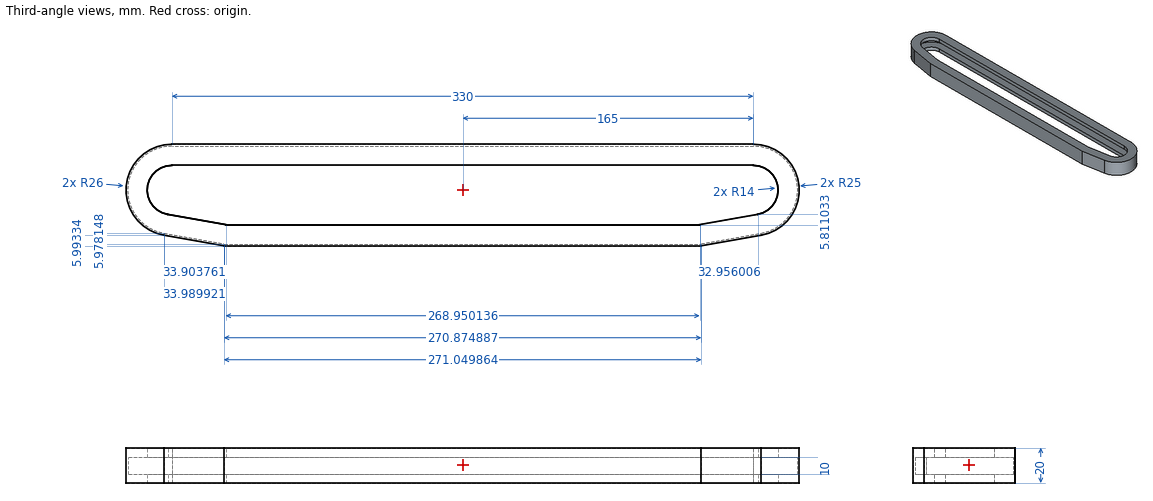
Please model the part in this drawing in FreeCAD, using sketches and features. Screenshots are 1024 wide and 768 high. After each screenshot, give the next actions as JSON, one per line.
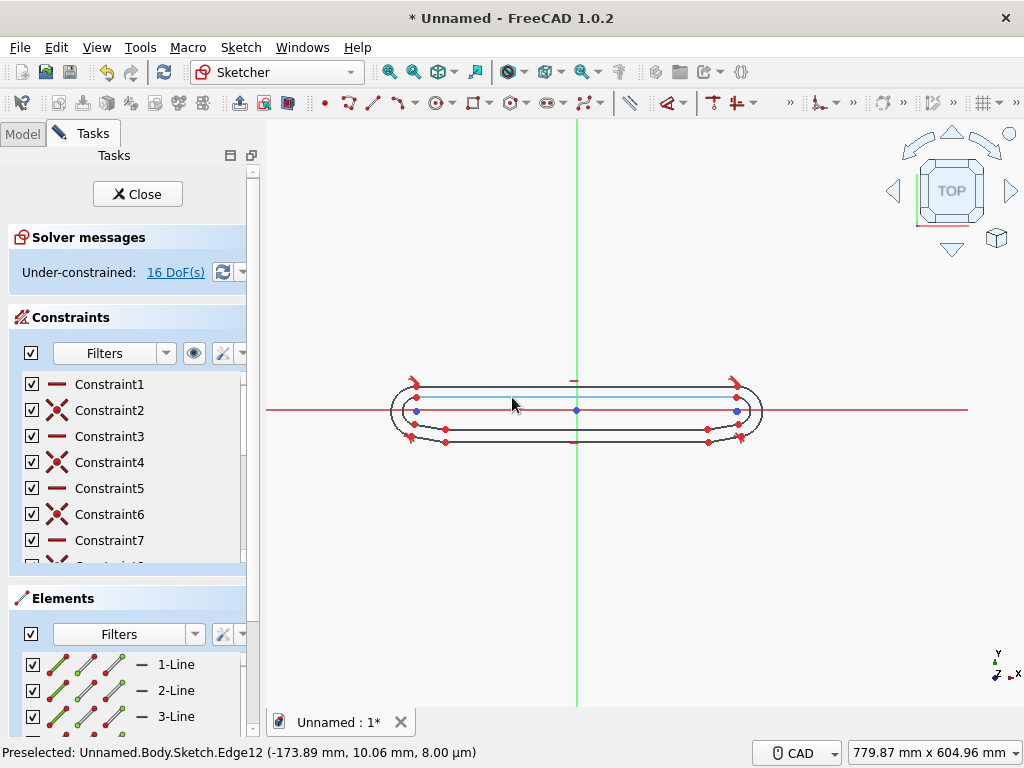
{"action": "left_click", "coordinate": [759, 424]}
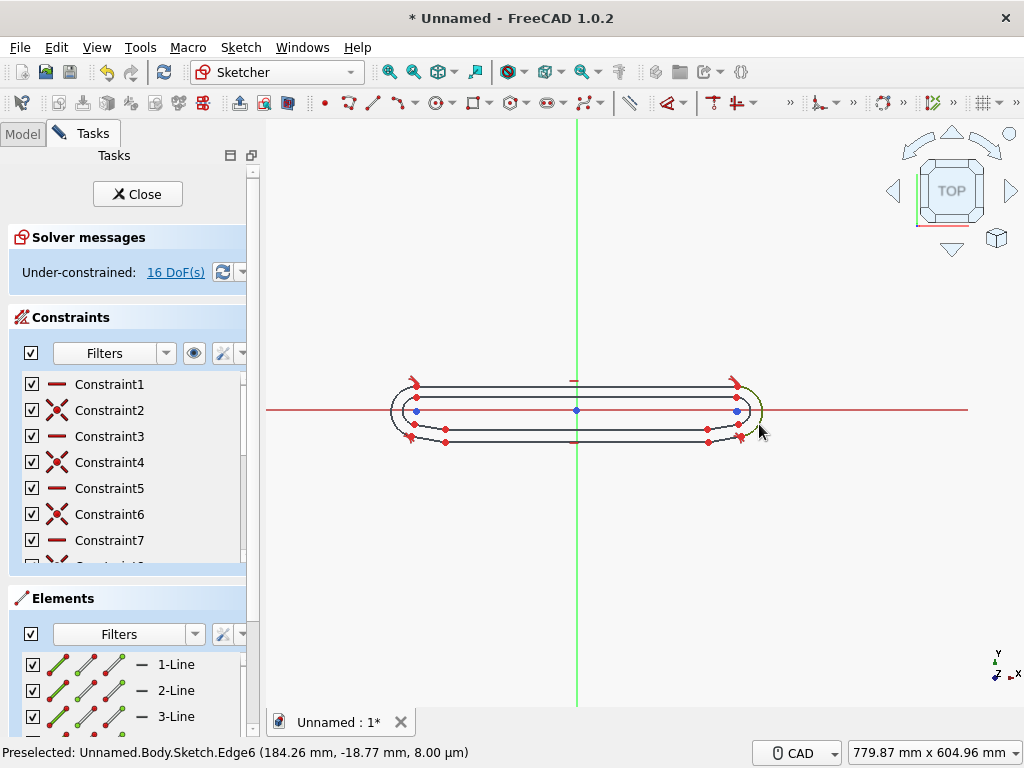
{"action": "left_click", "coordinate": [750, 410]}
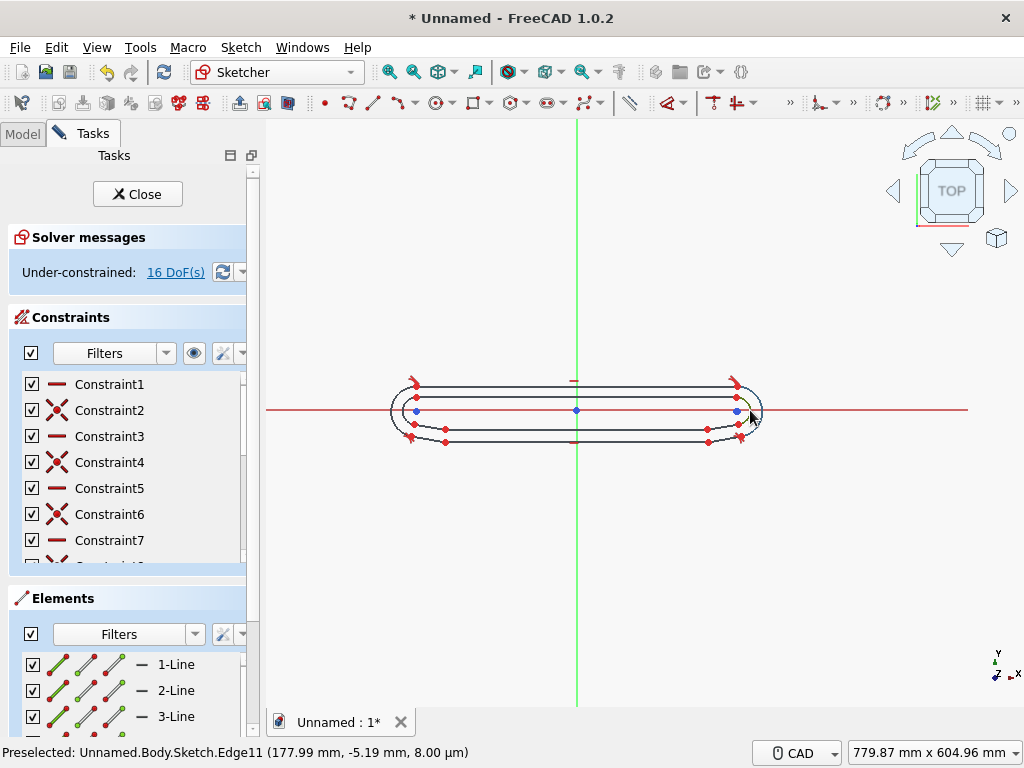
{"action": "left_click", "coordinate": [714, 104]}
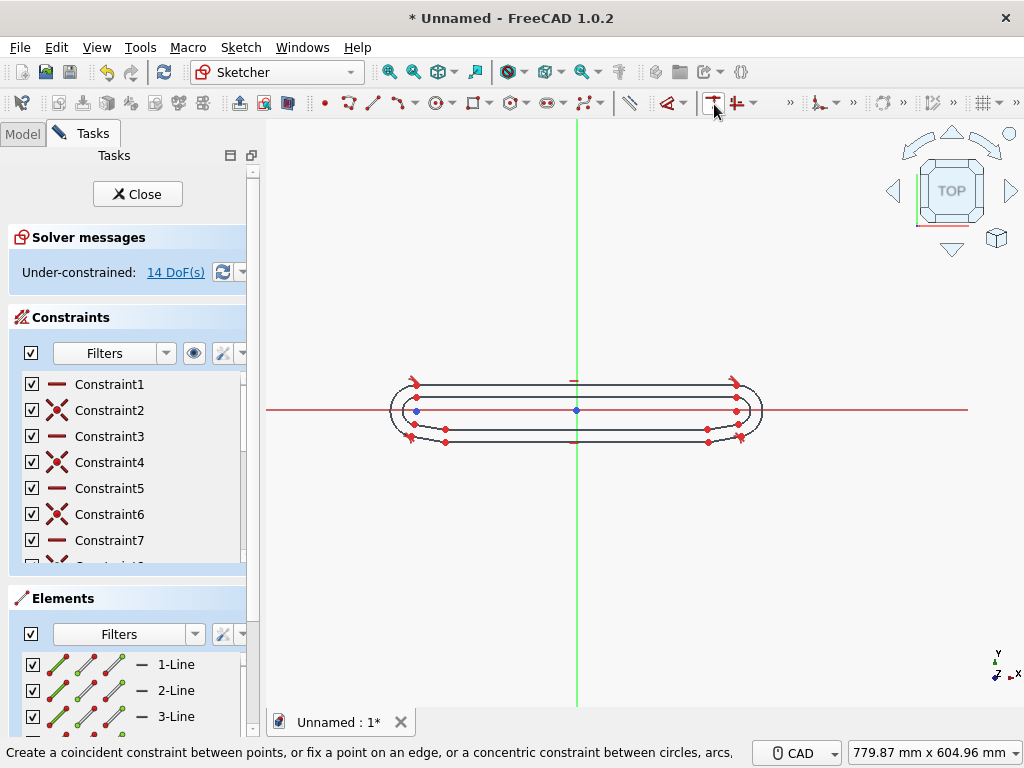
{"action": "left_click", "coordinate": [396, 395]}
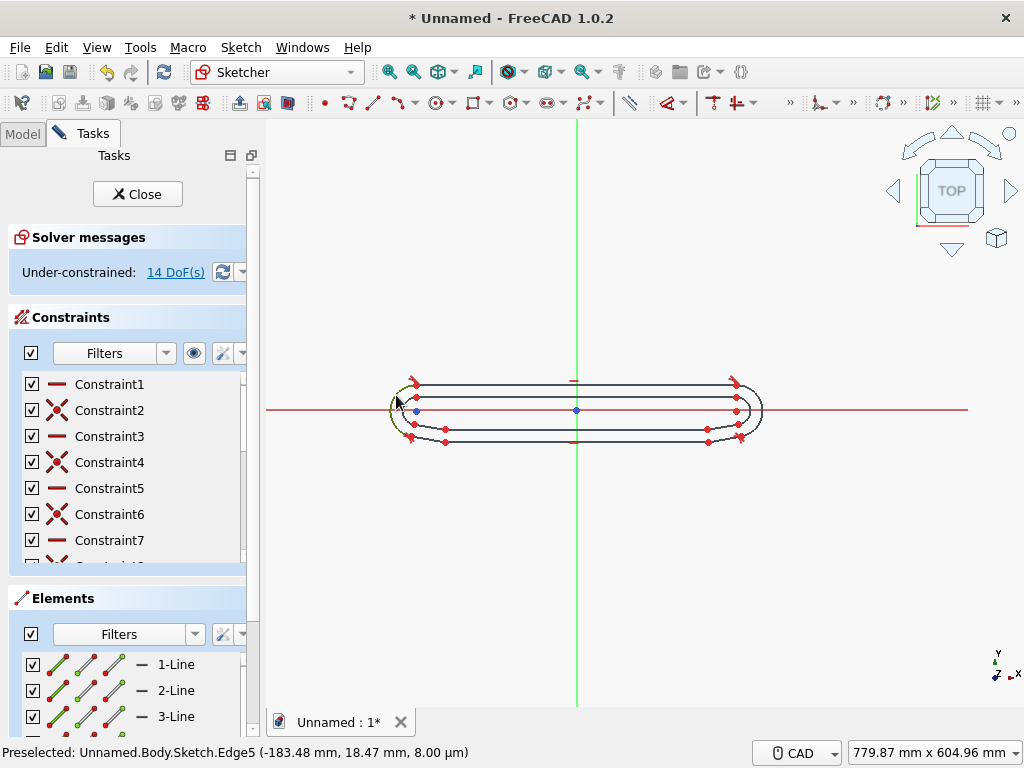
{"action": "left_click", "coordinate": [403, 410]}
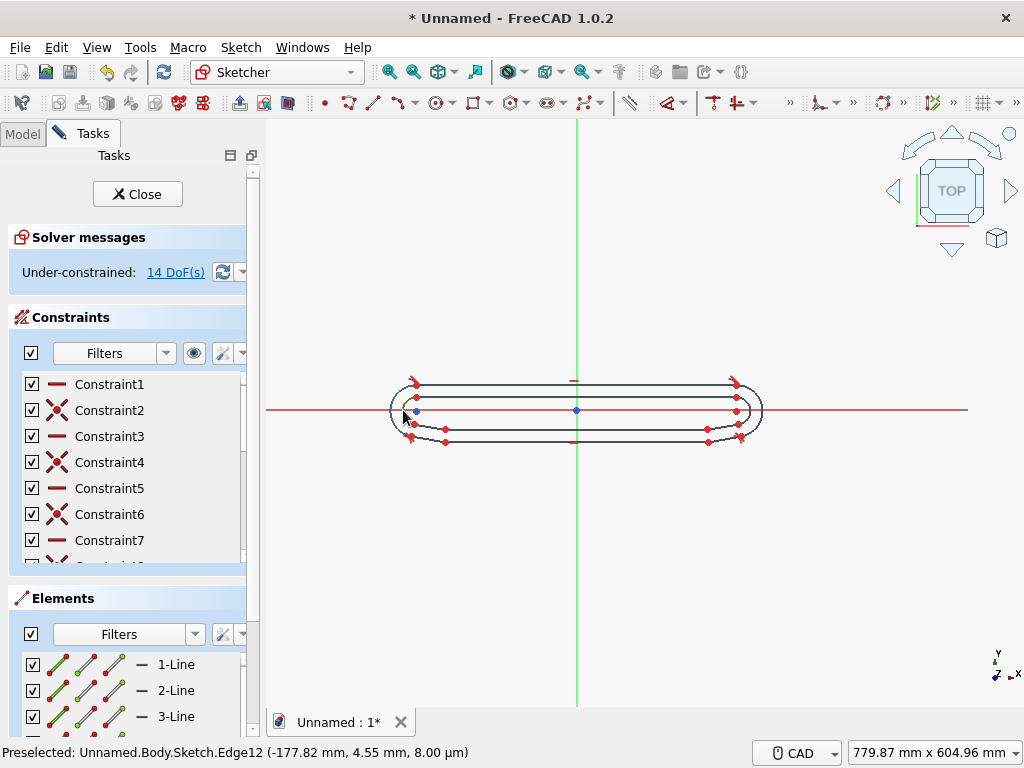
{"action": "left_click", "coordinate": [714, 104]}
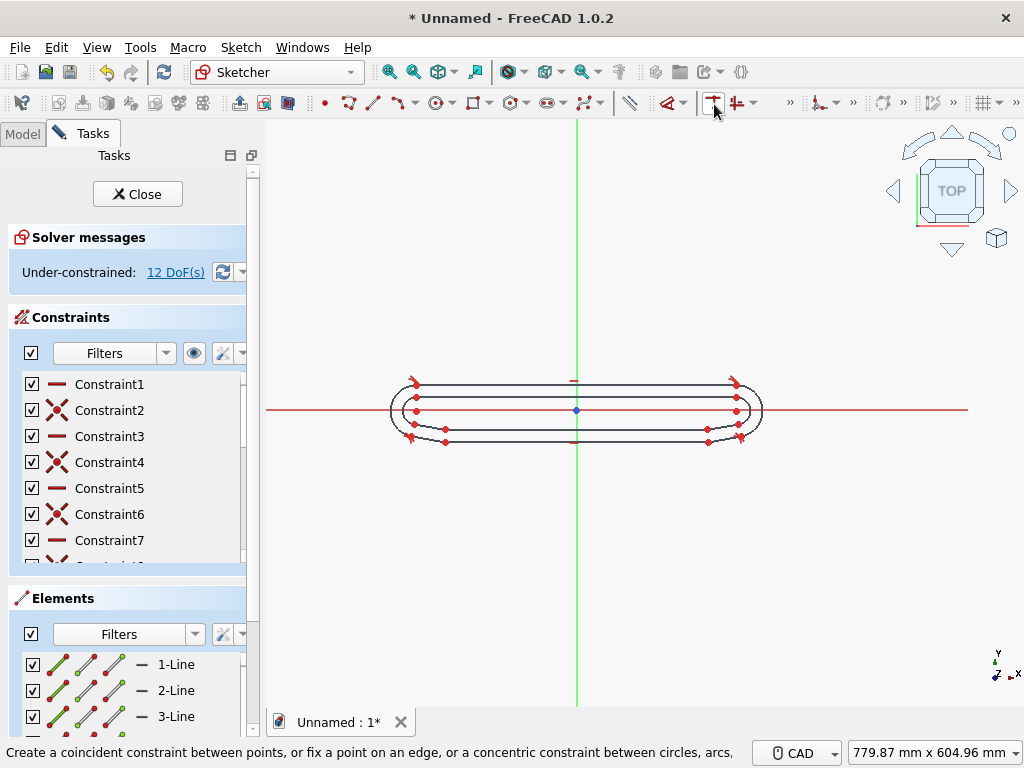
{"action": "left_click", "coordinate": [396, 395]}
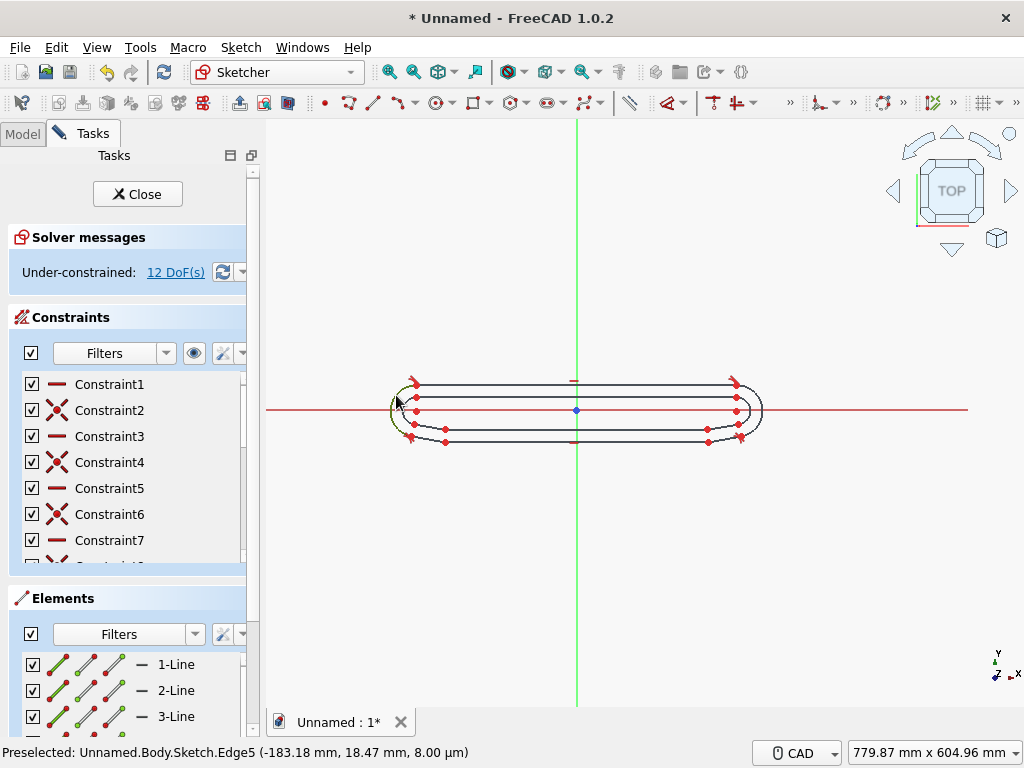
{"action": "left_click", "coordinate": [759, 424]}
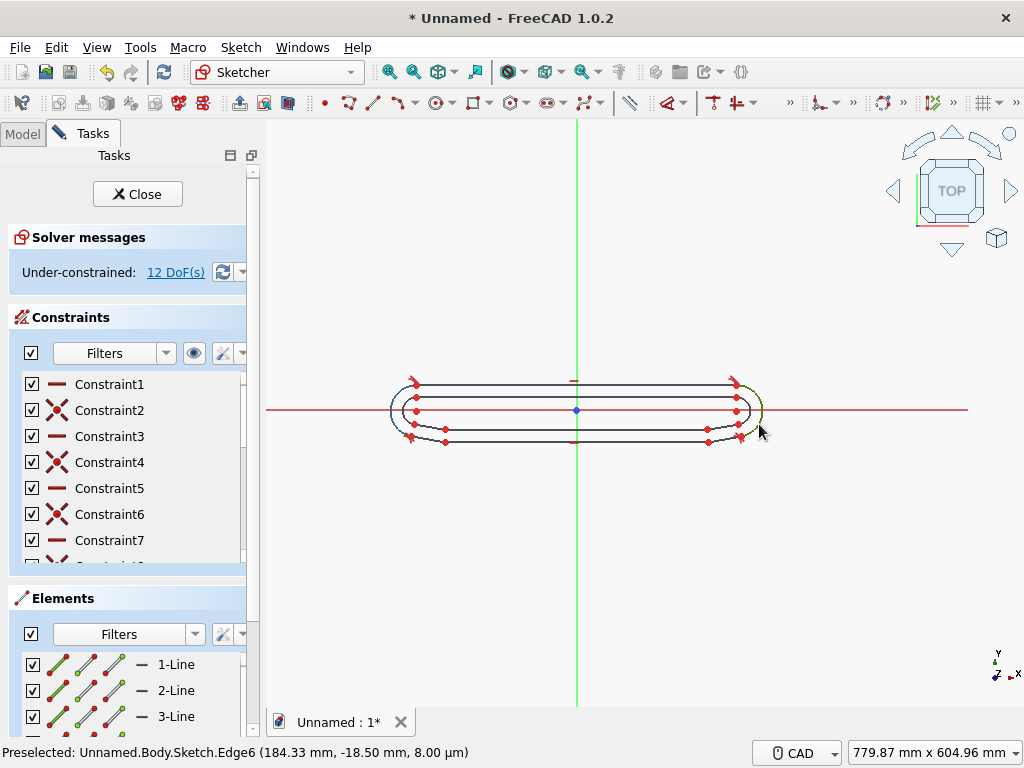
{"action": "key", "text": "e"}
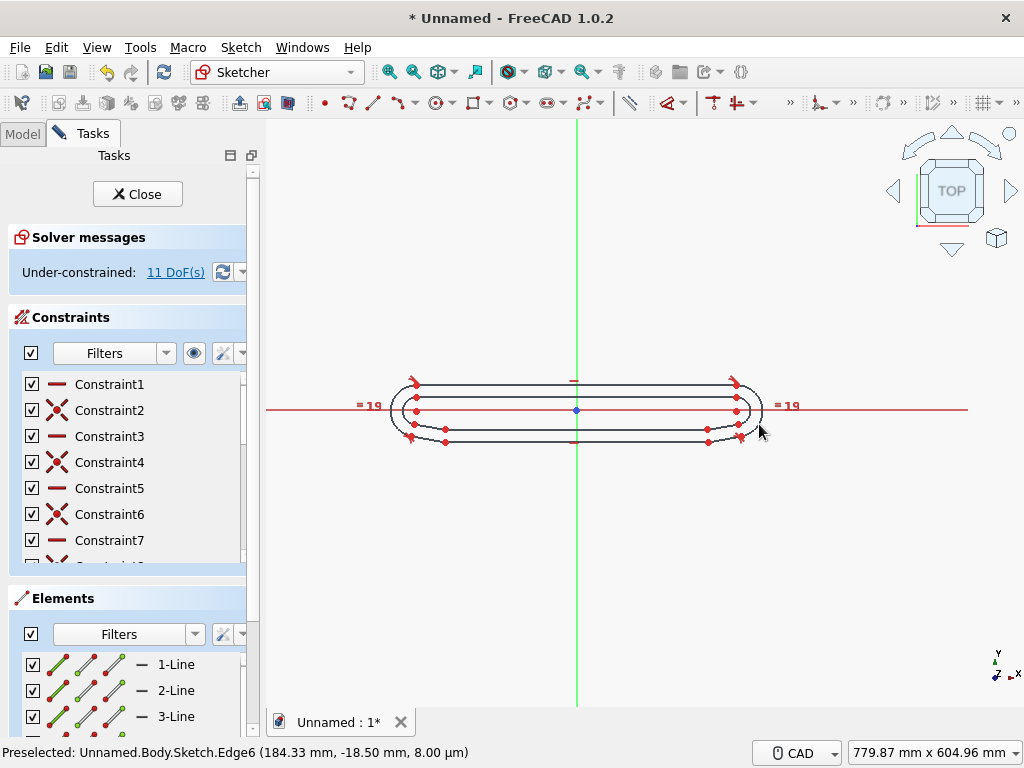
{"action": "left_click", "coordinate": [417, 411]}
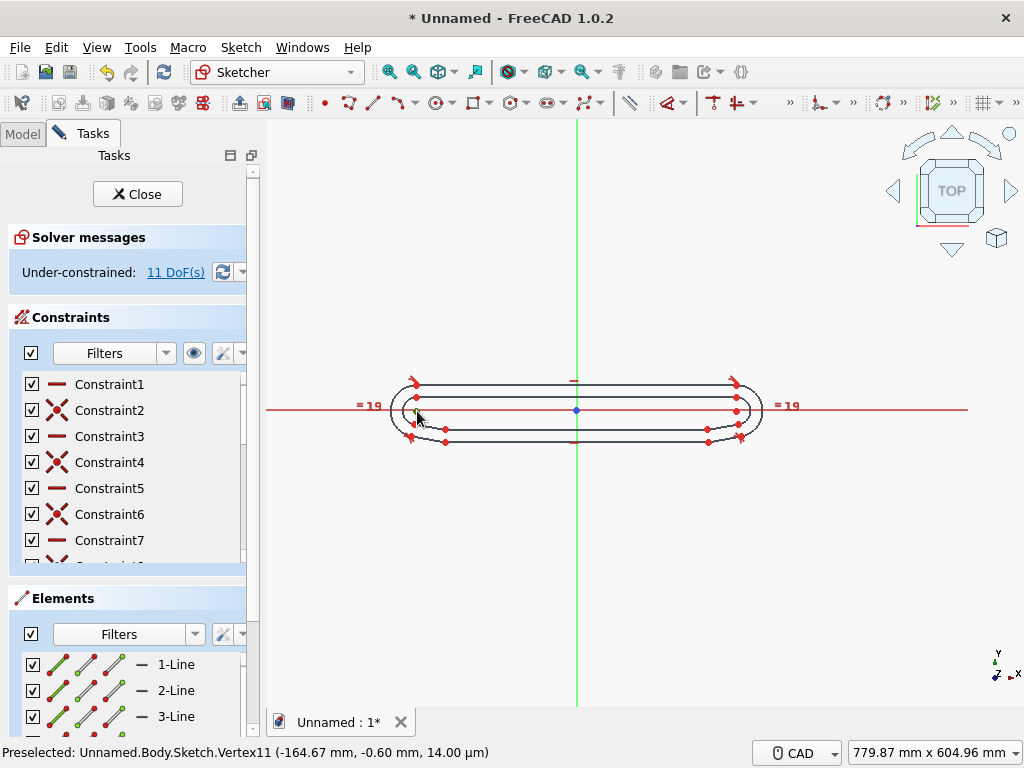
{"action": "left_click", "coordinate": [334, 410]}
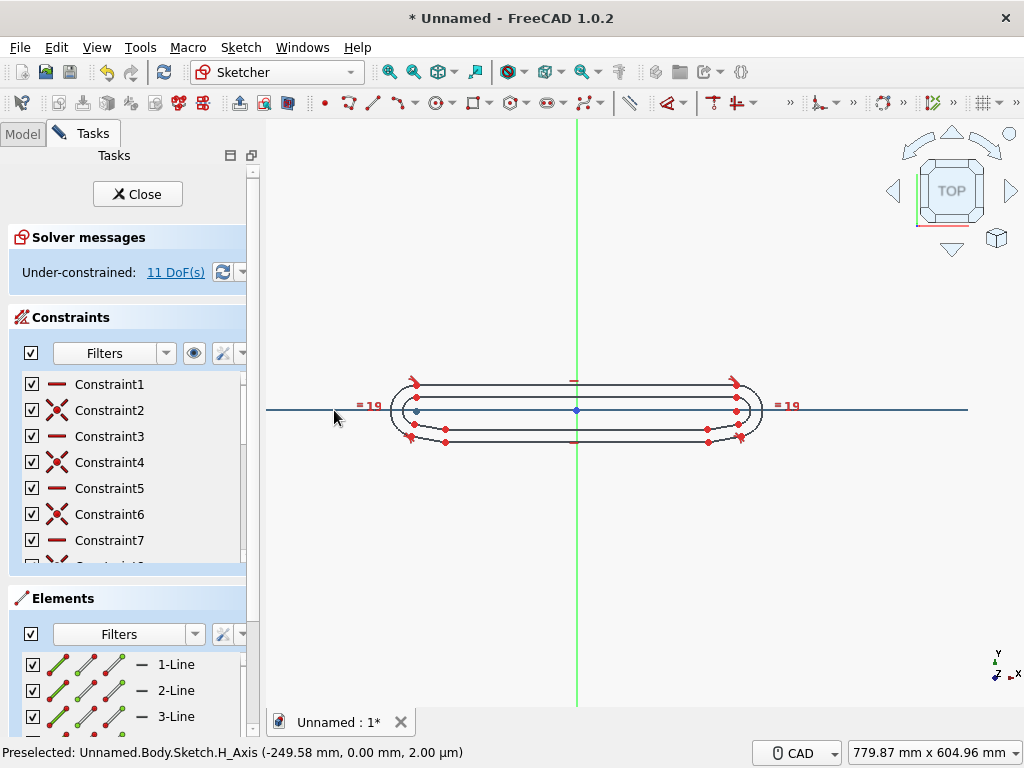
{"action": "left_click", "coordinate": [714, 104]}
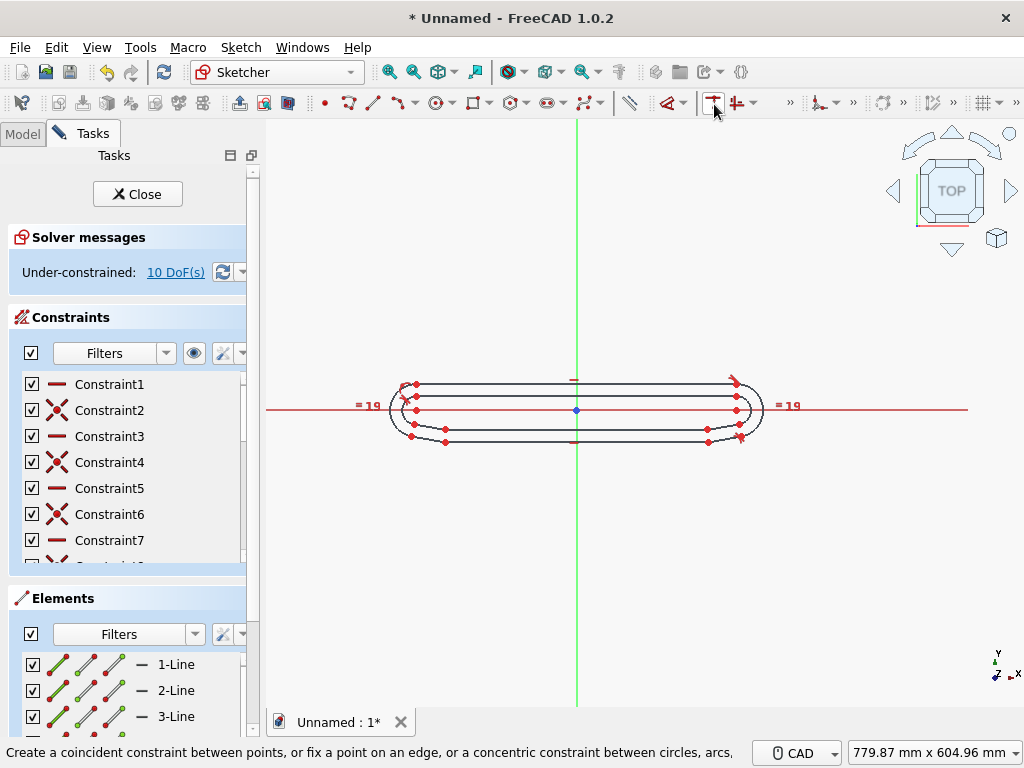
{"action": "left_click", "coordinate": [668, 104]}